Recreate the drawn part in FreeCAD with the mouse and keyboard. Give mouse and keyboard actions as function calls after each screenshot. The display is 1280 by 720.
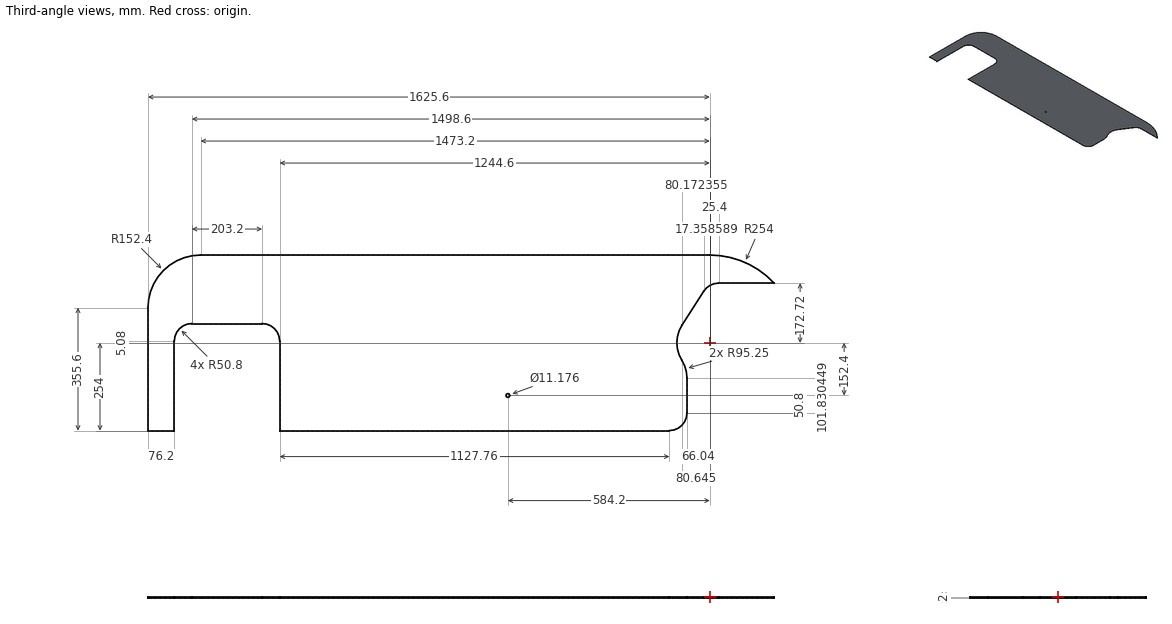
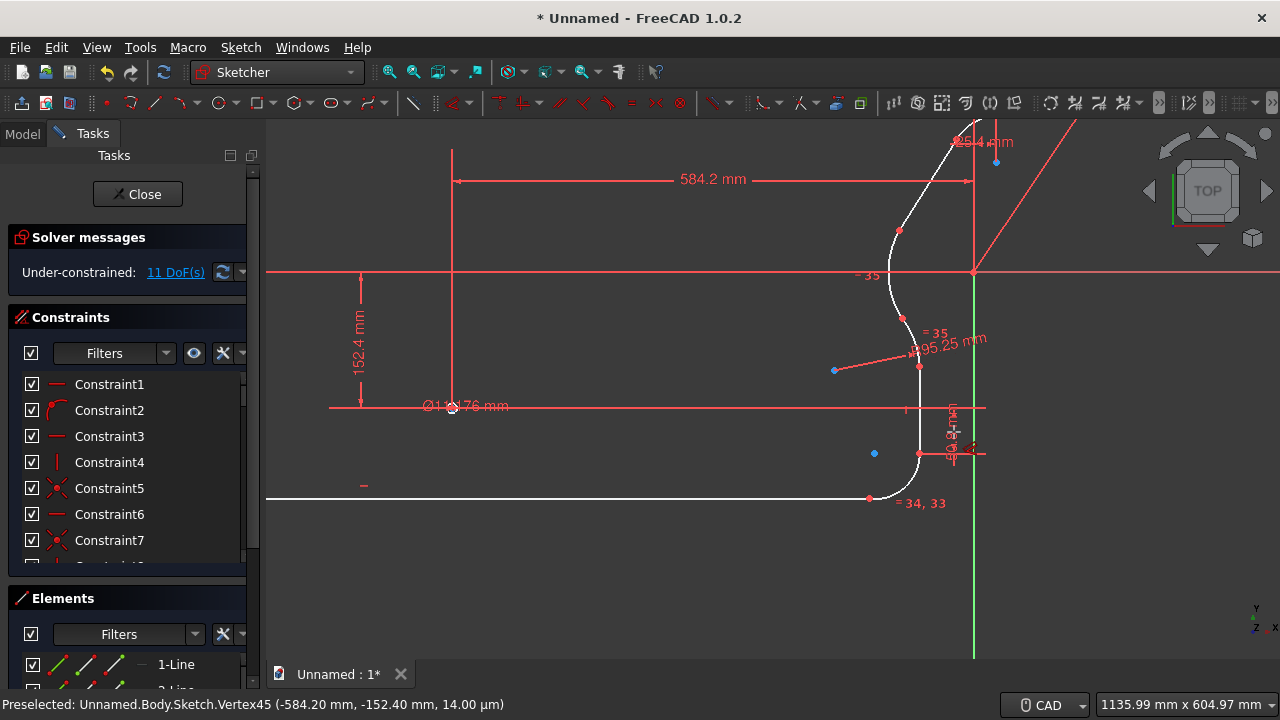
scroll(922, 457, down, 5)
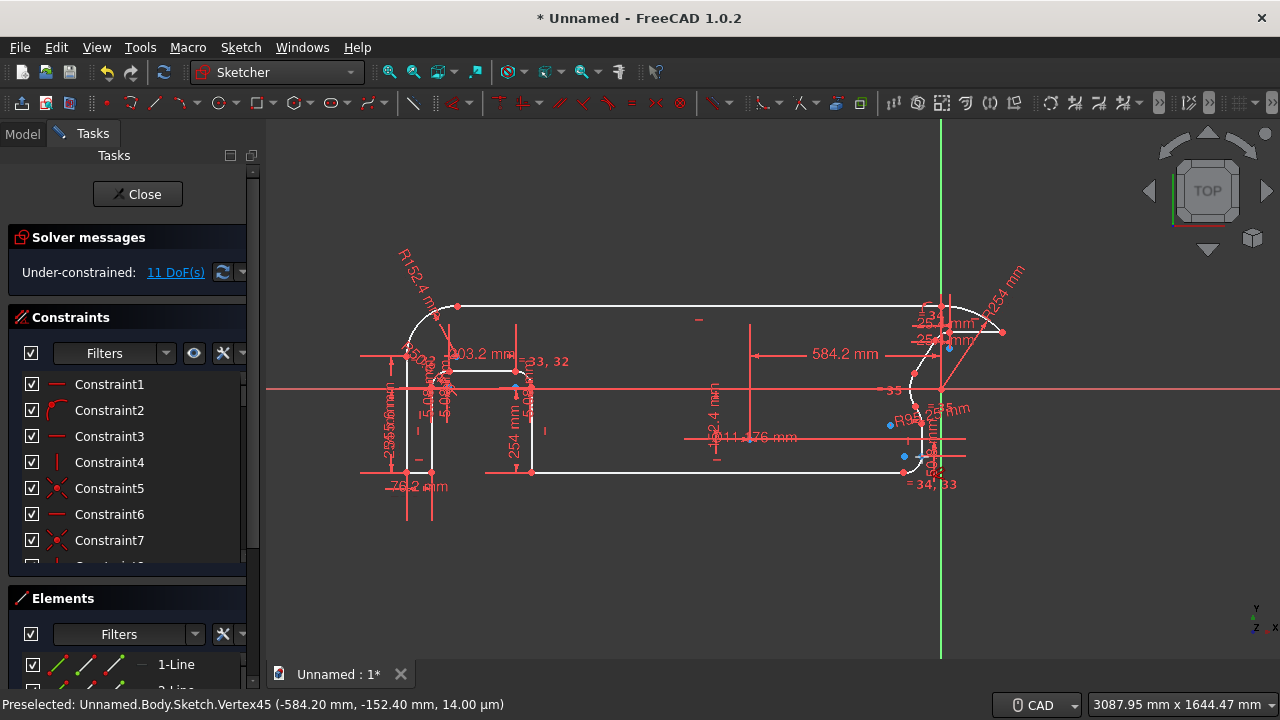
click(796, 306)
click(699, 272)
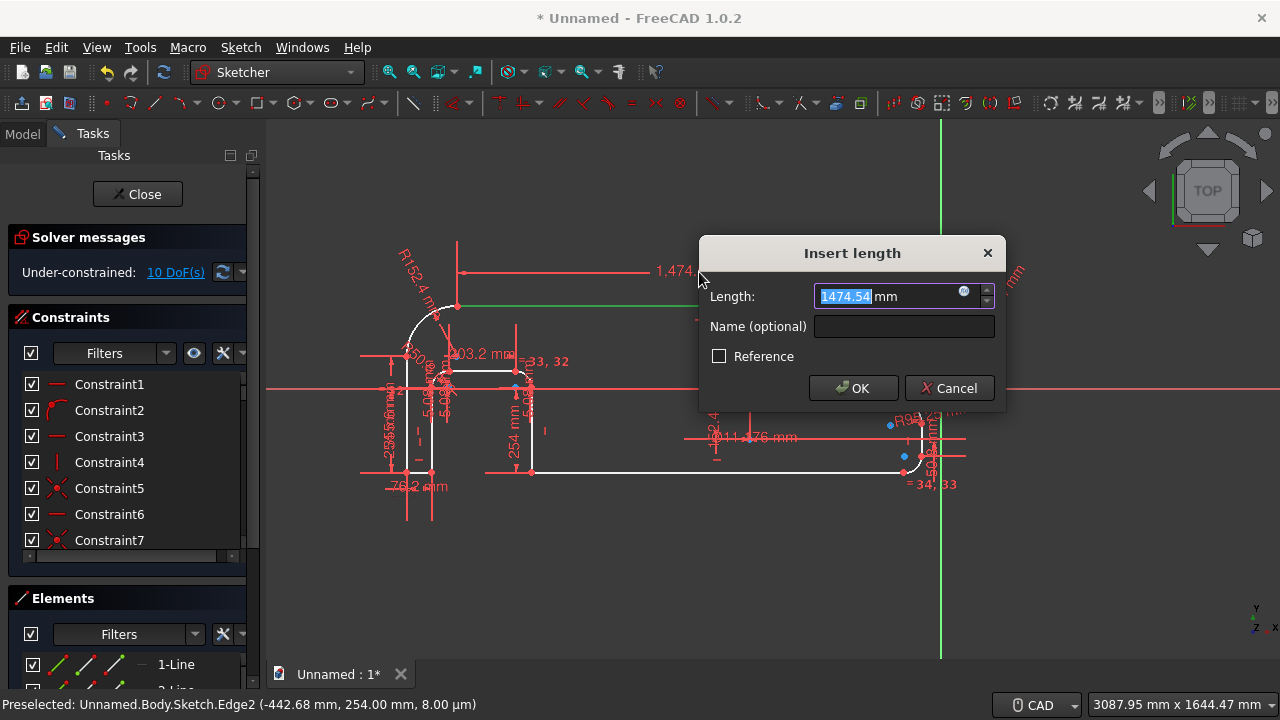
text(1473.2)
key(Return)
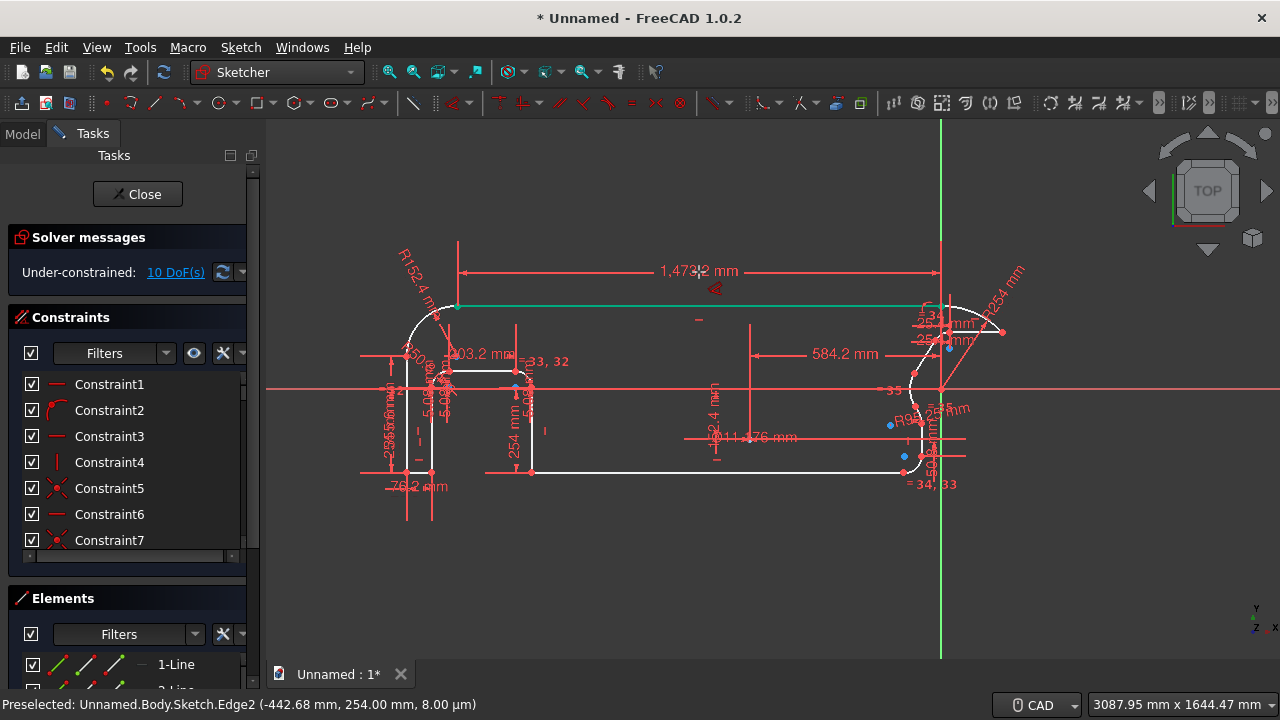
scroll(922, 456, up, 4)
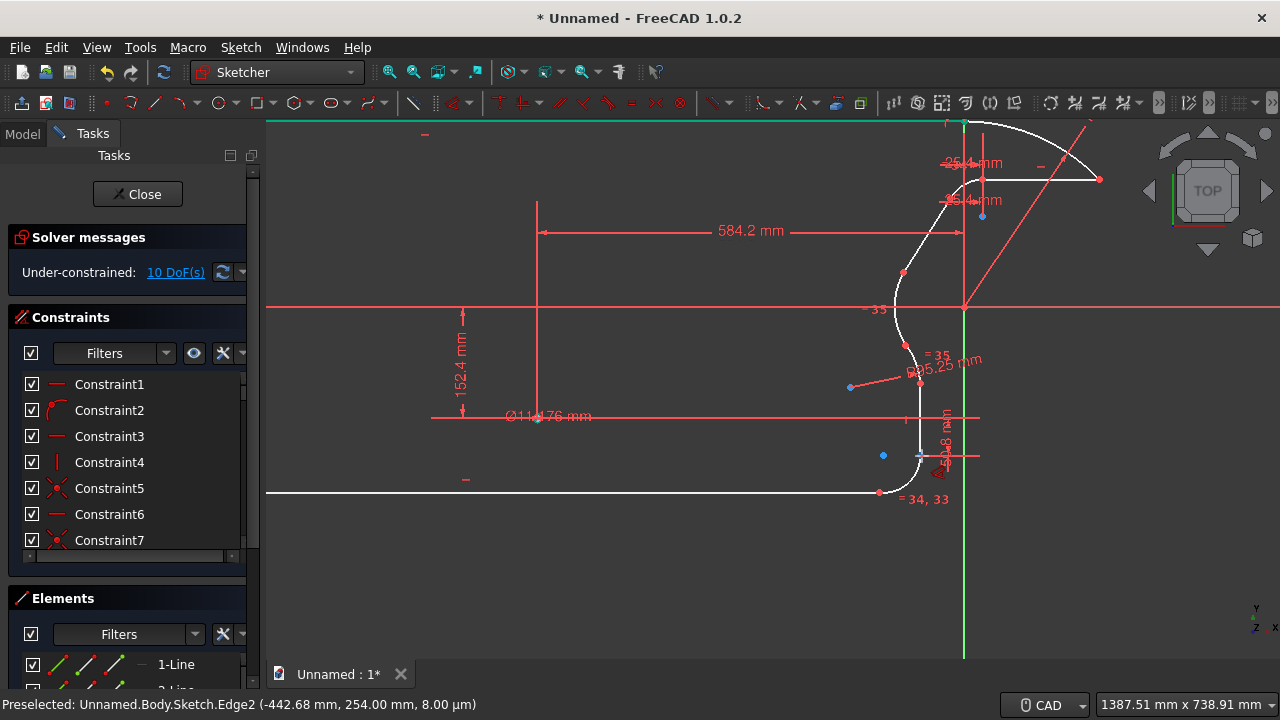
click(920, 456)
click(942, 490)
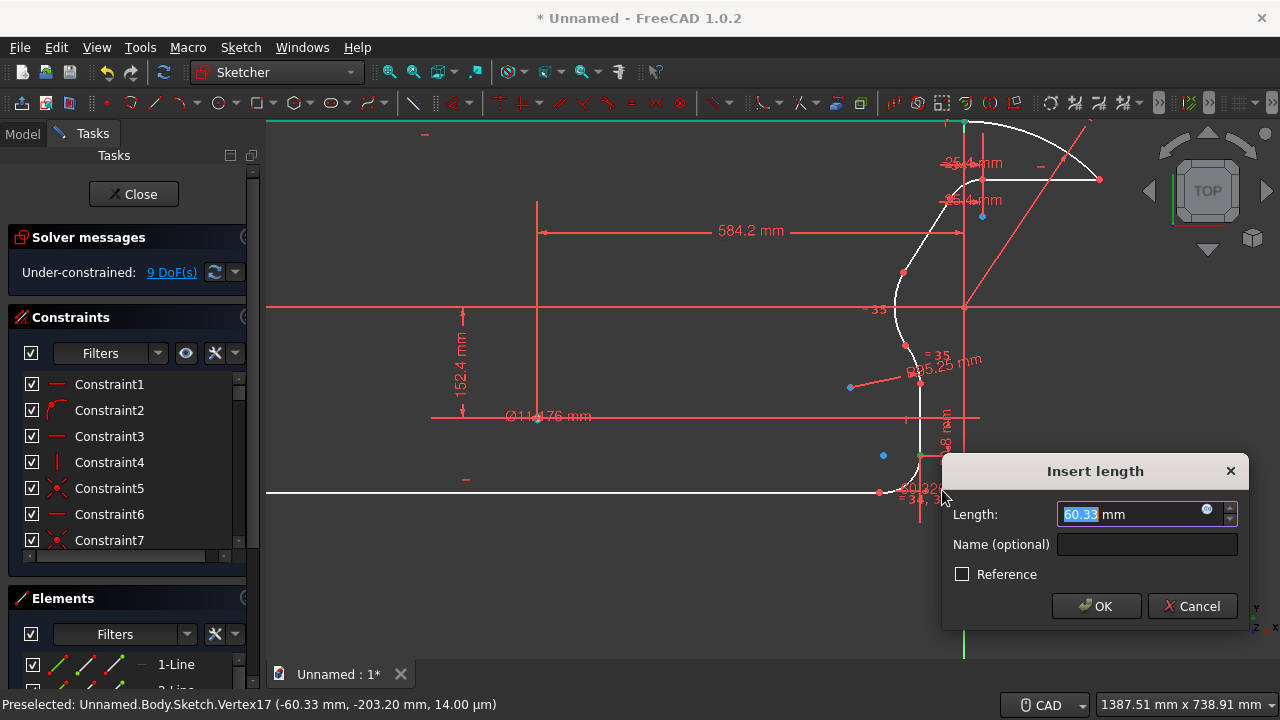
text(66.04)
key(Return)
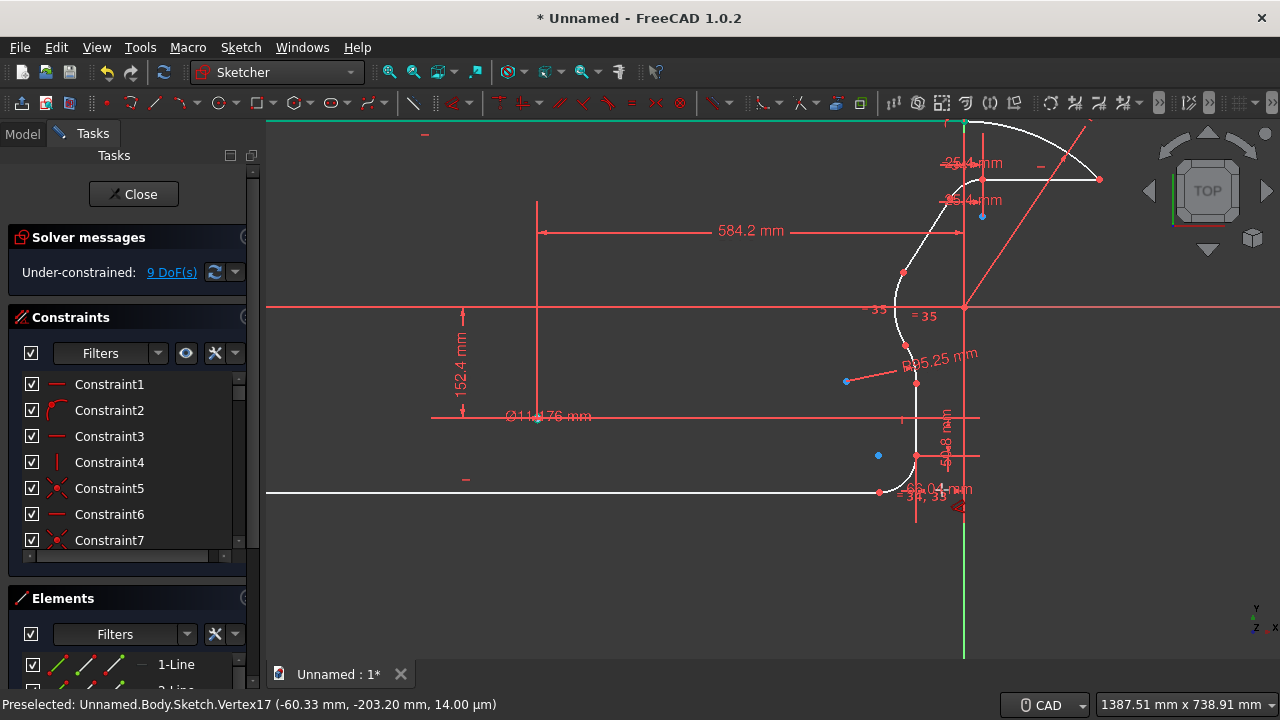
click(301, 493)
click(587, 527)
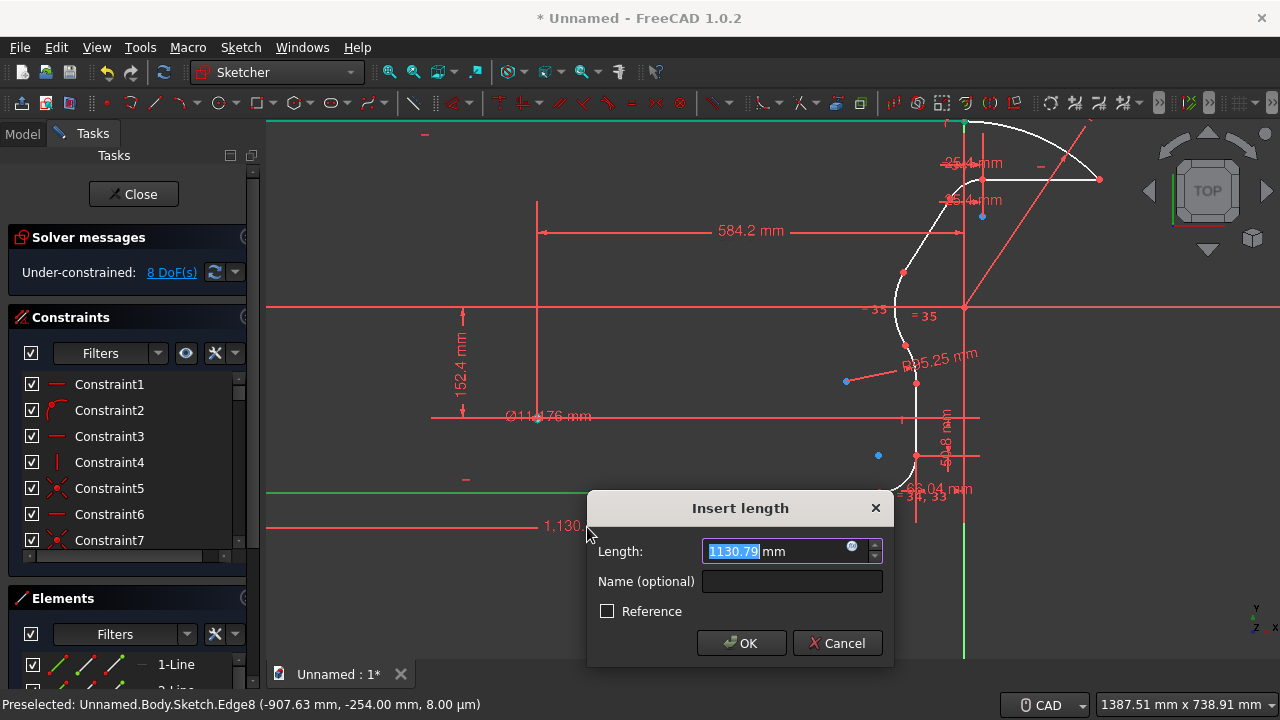
text(1127.76)
key(Return)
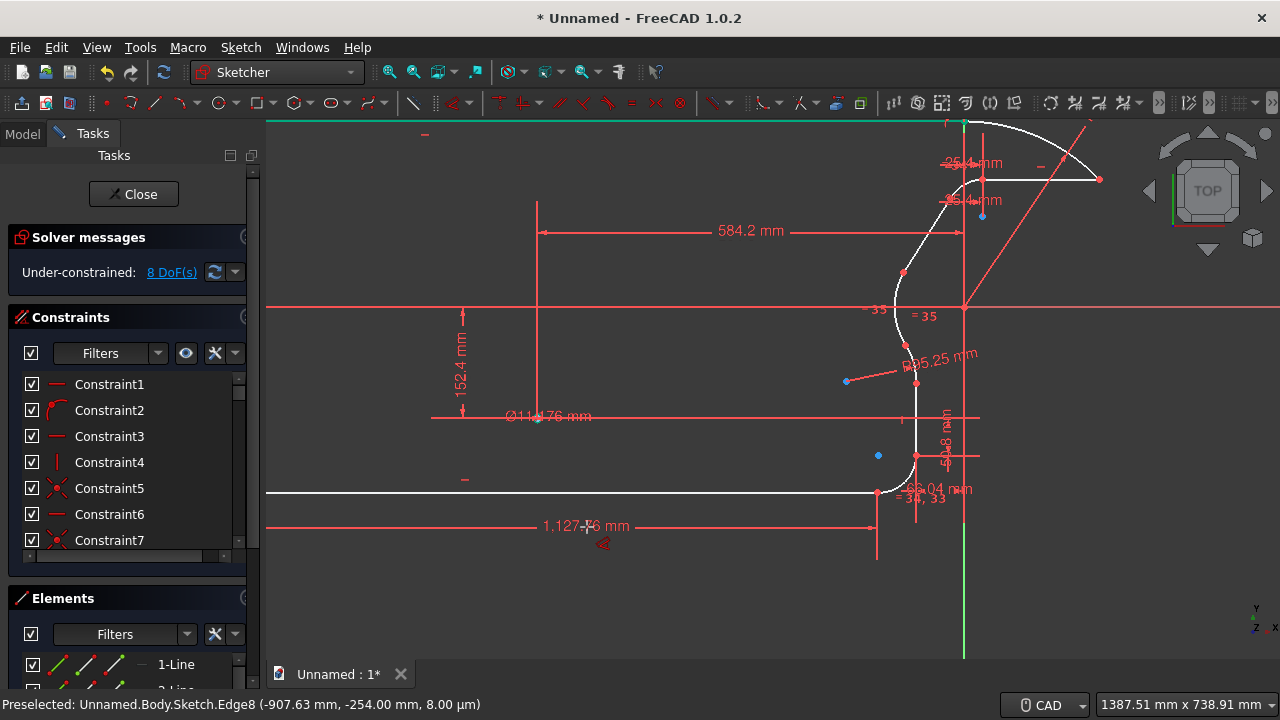
click(983, 180)
click(1017, 243)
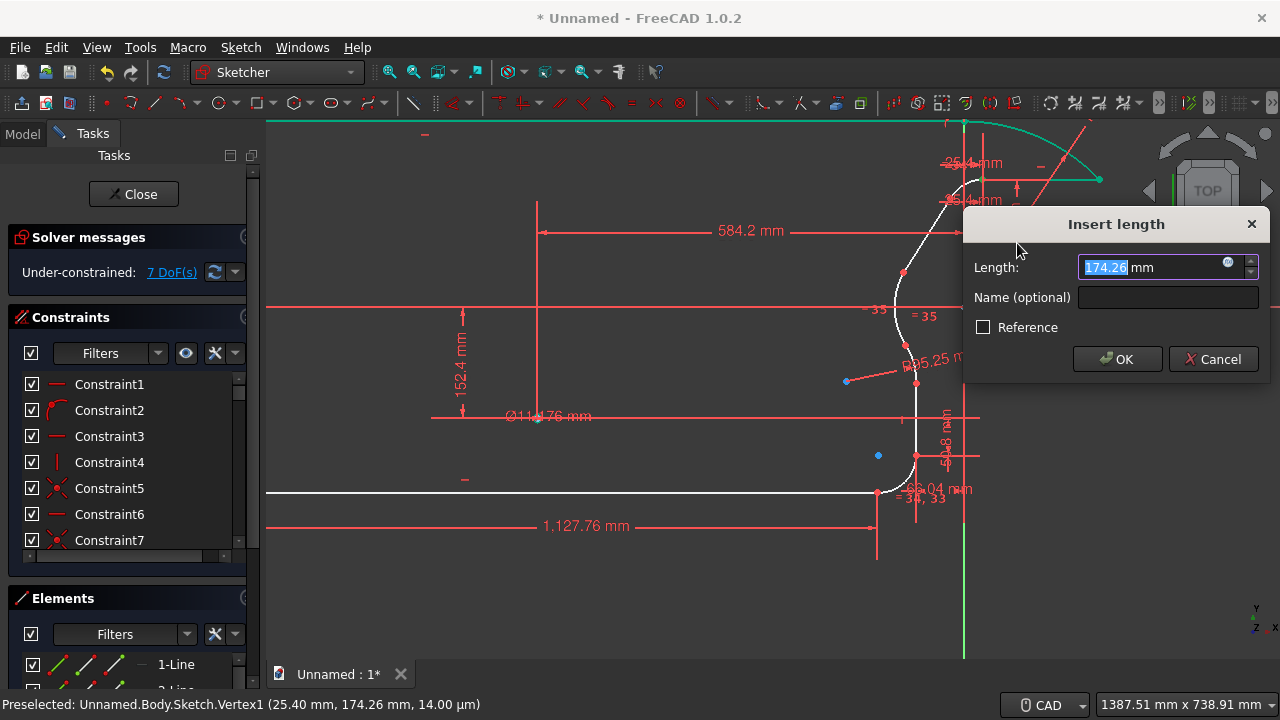
text(172.72)
key(Return)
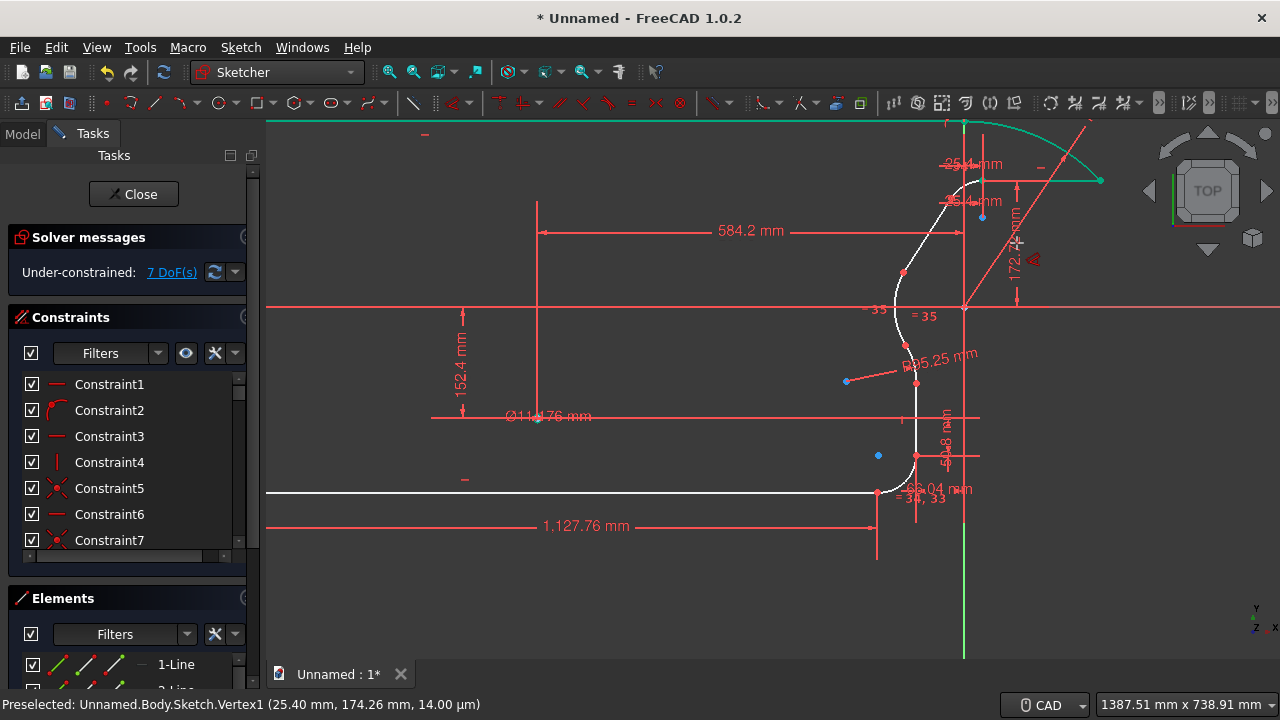
scroll(922, 456, down, 4)